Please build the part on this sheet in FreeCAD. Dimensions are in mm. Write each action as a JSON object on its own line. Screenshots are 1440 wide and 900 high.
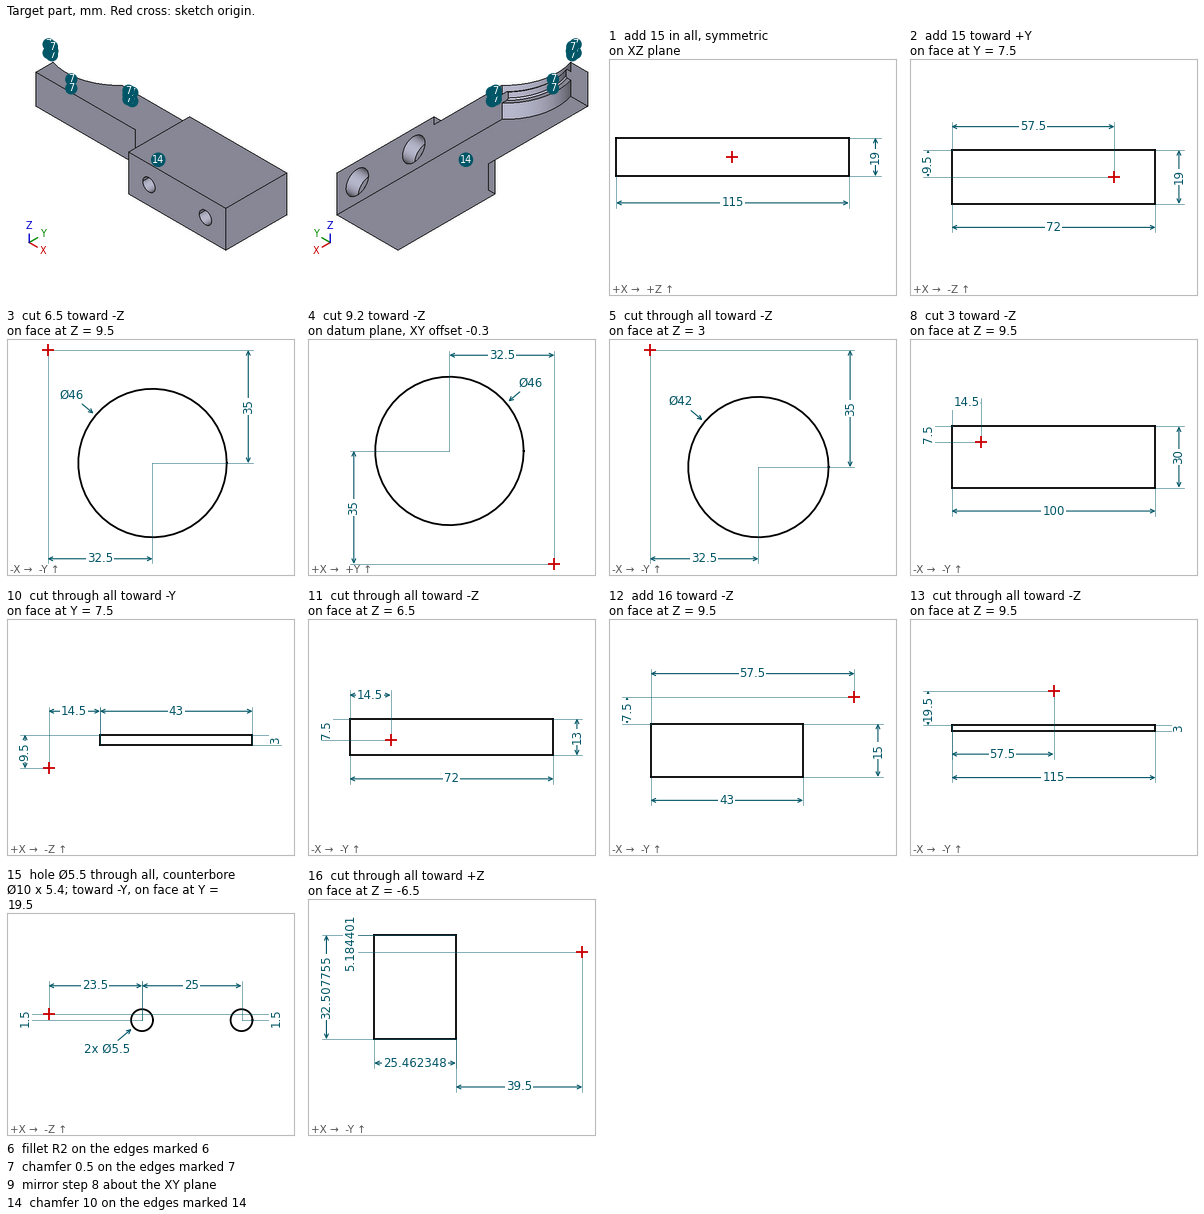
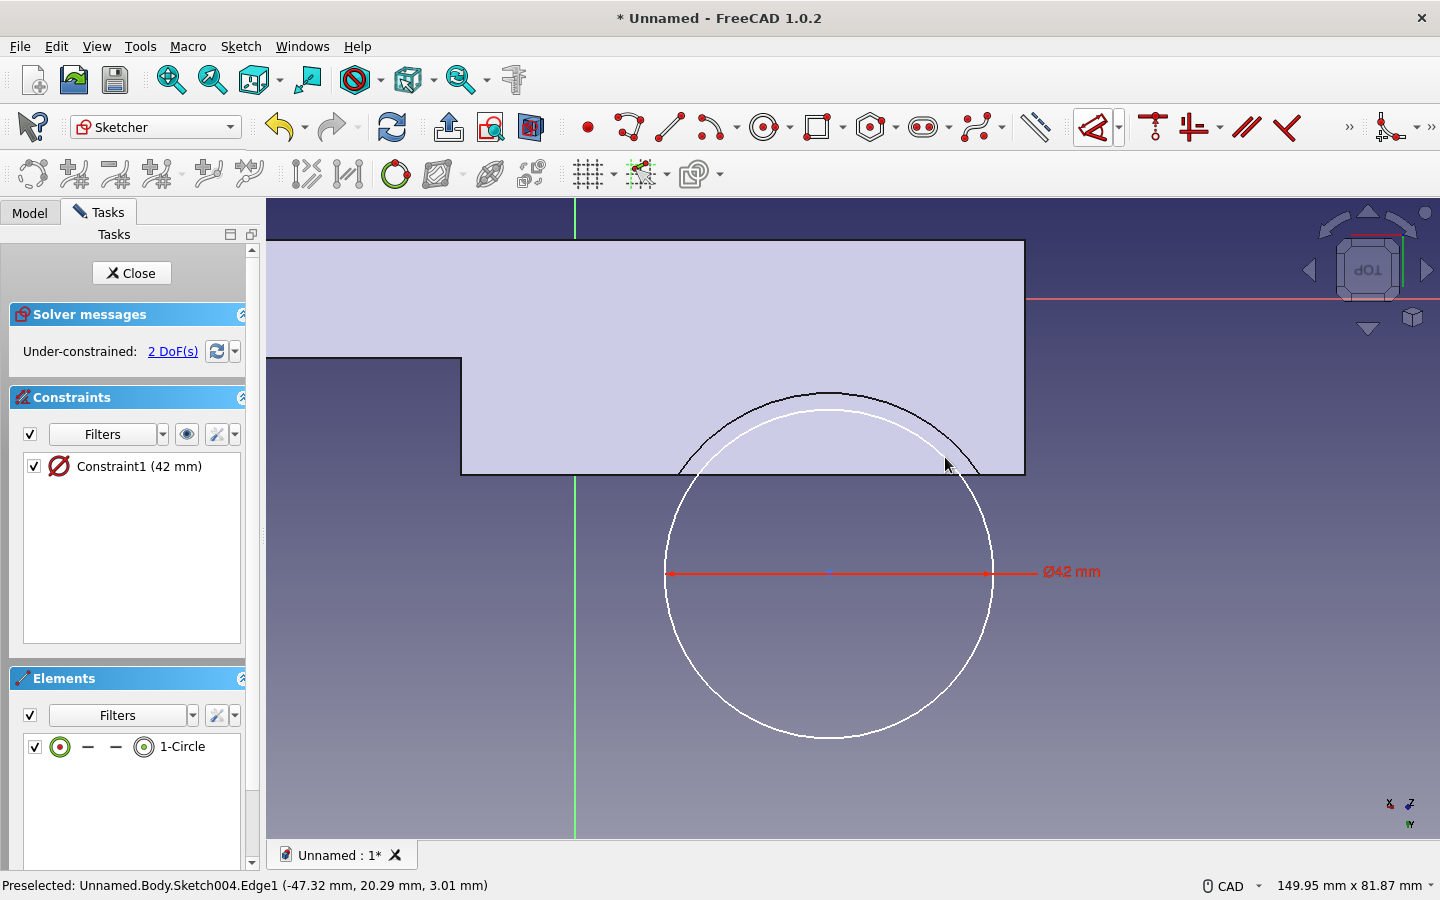
{"action": "left_click", "coordinate": [829, 574]}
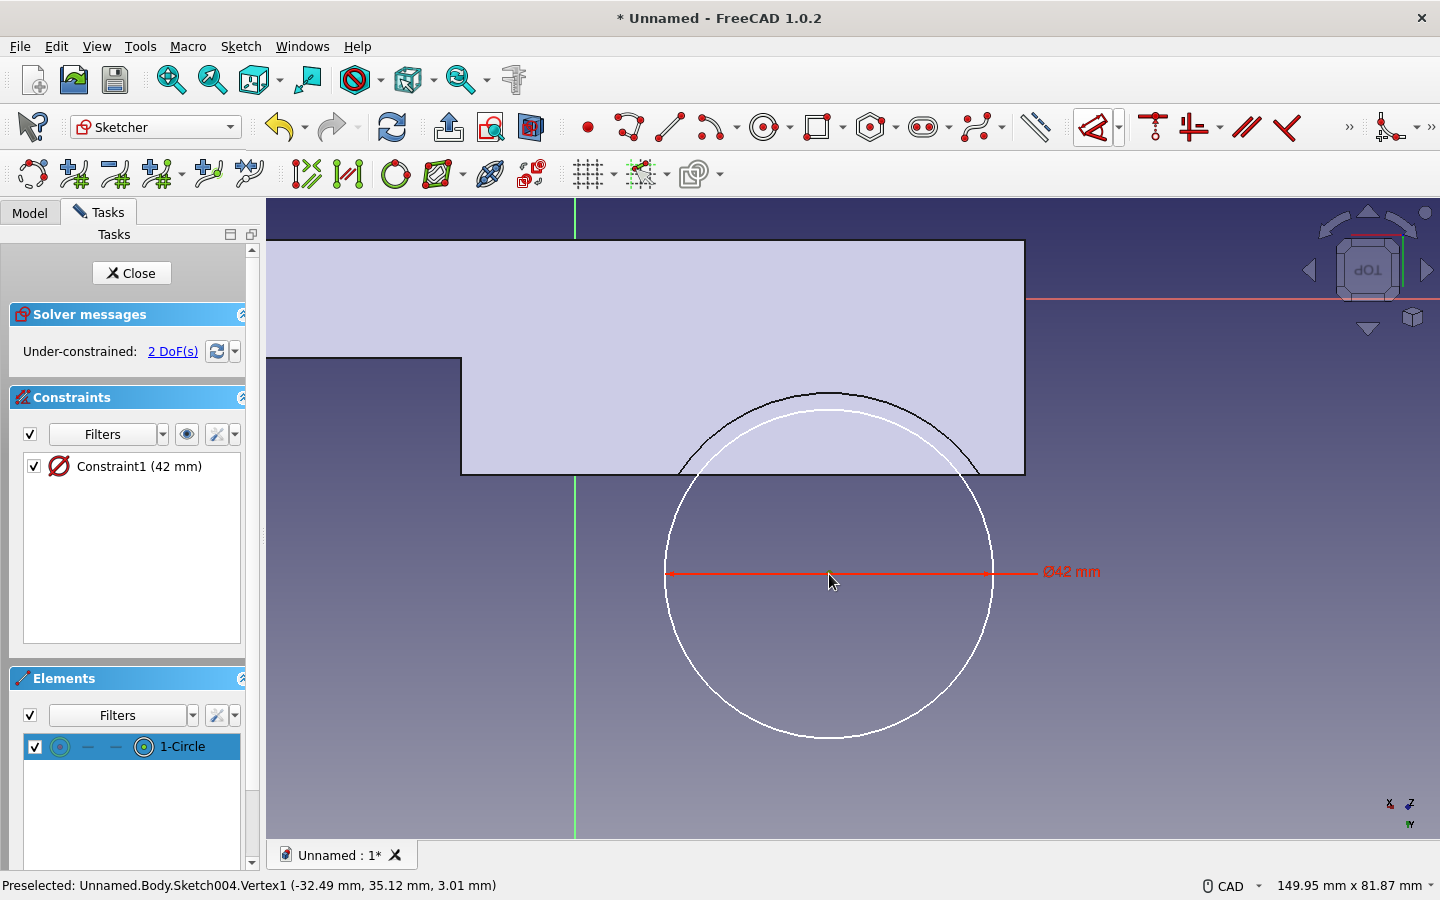
{"action": "left_click", "coordinate": [1118, 128]}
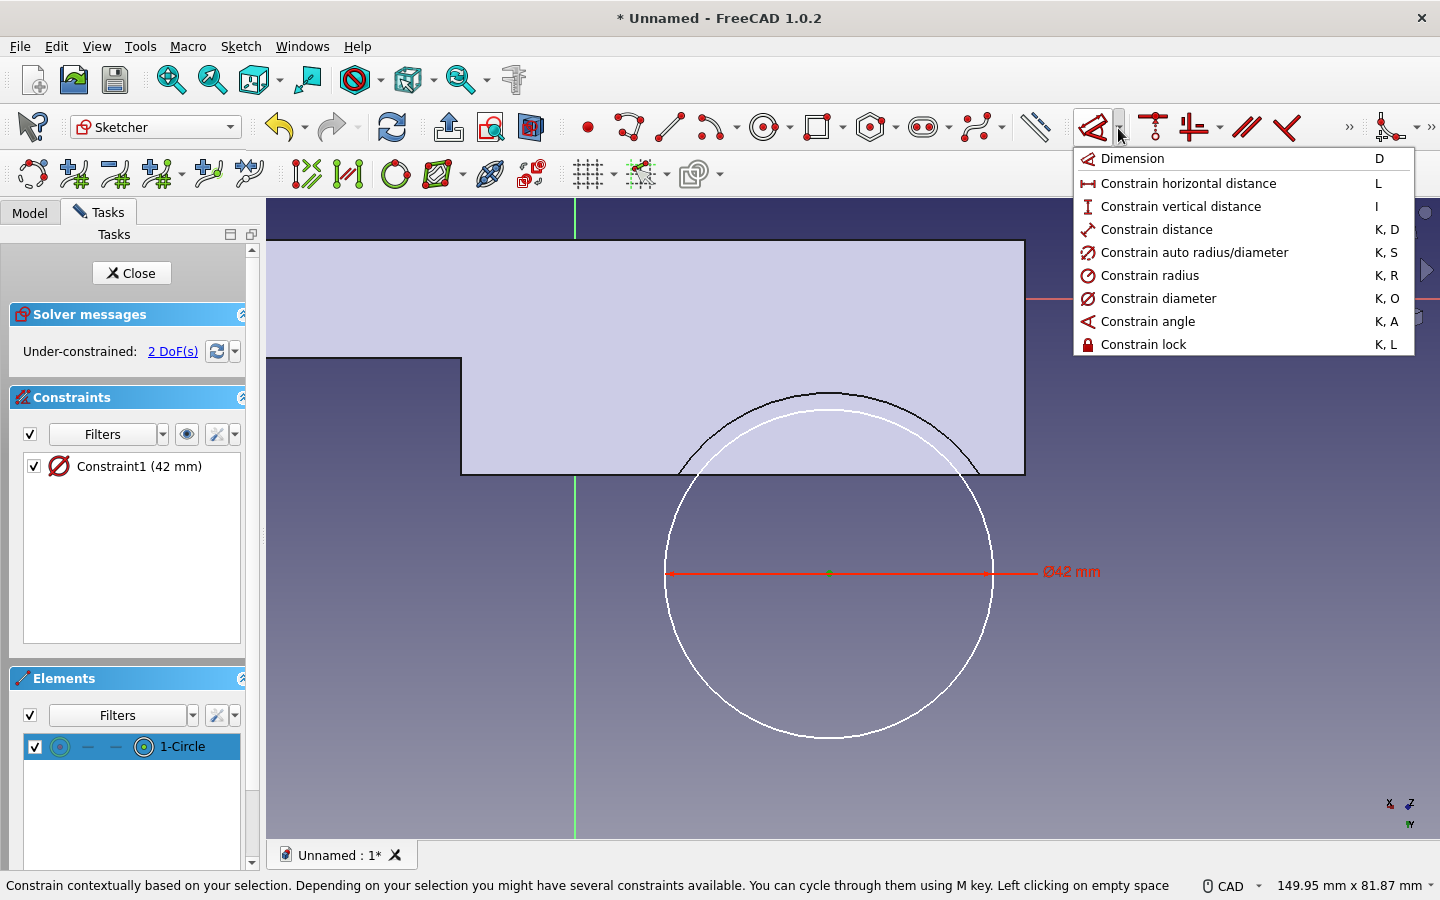
{"action": "left_click", "coordinate": [1244, 206]}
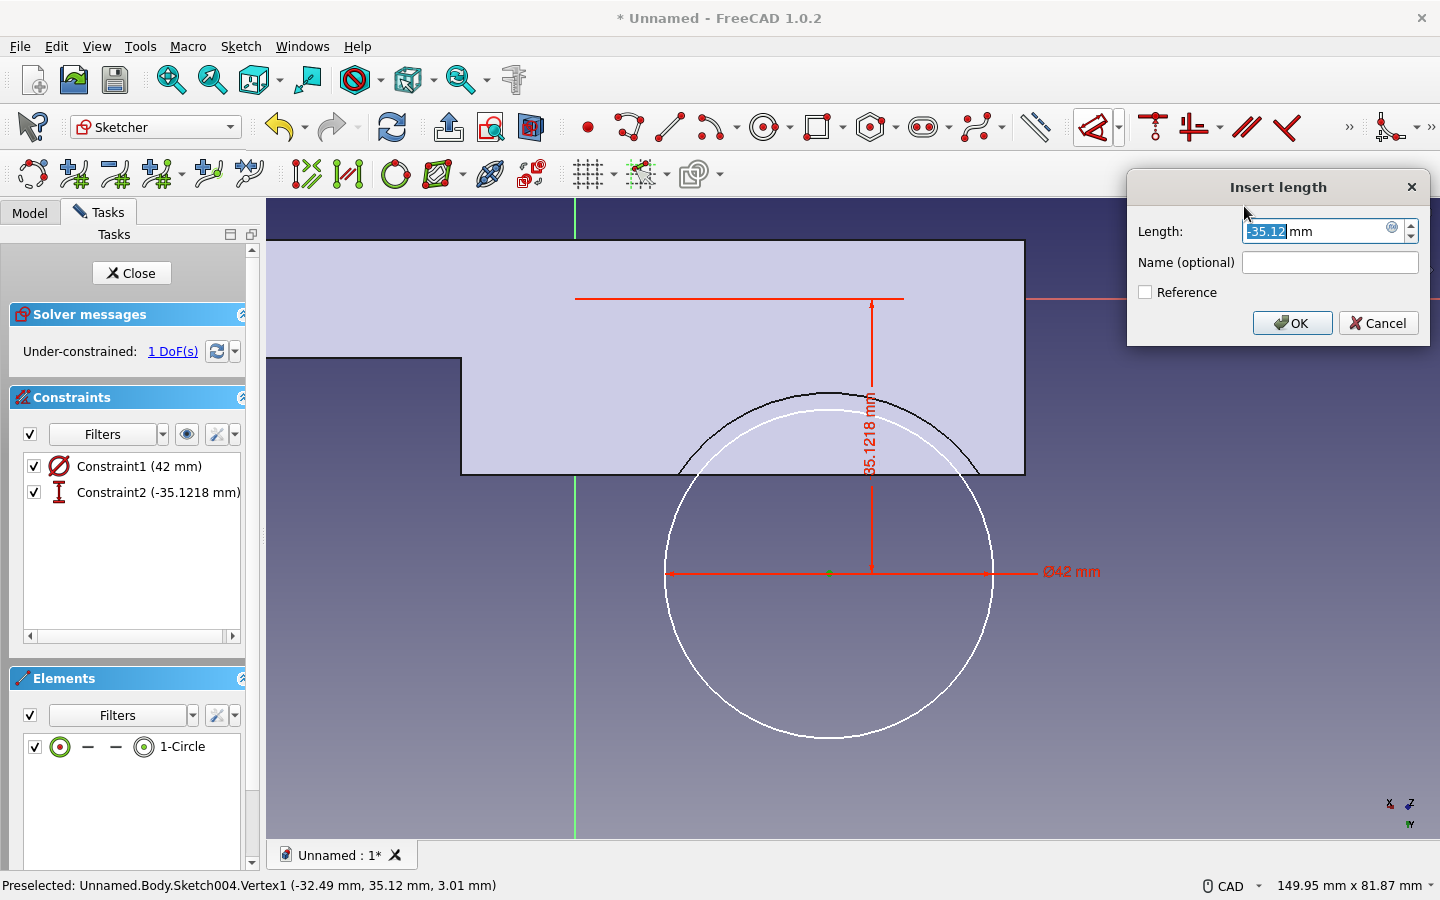
{"action": "type", "text": "-35"}
{"action": "key", "text": "Return"}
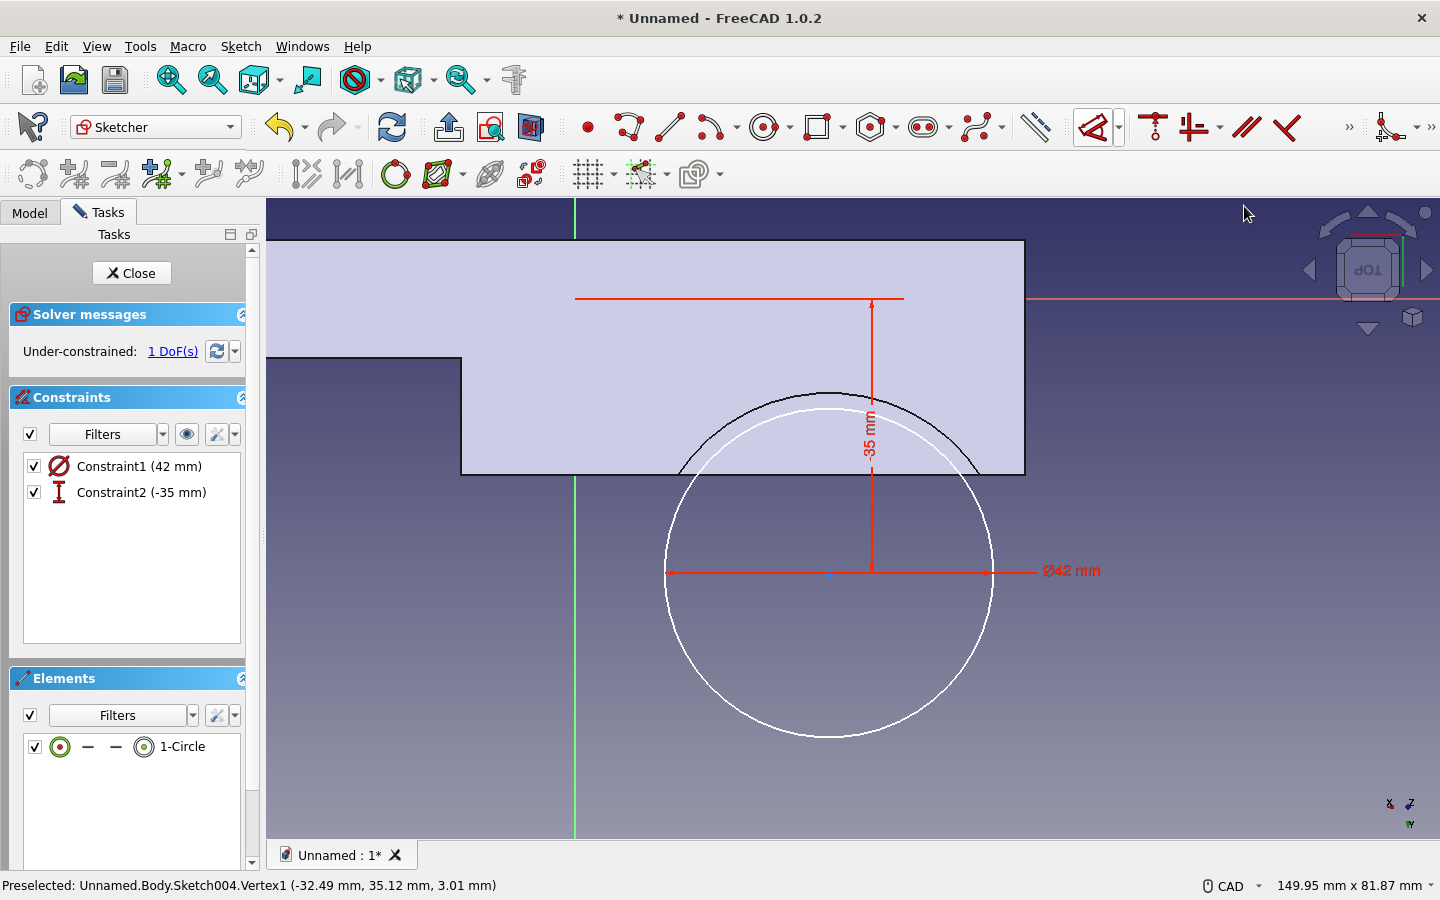
{"action": "left_click", "coordinate": [829, 573]}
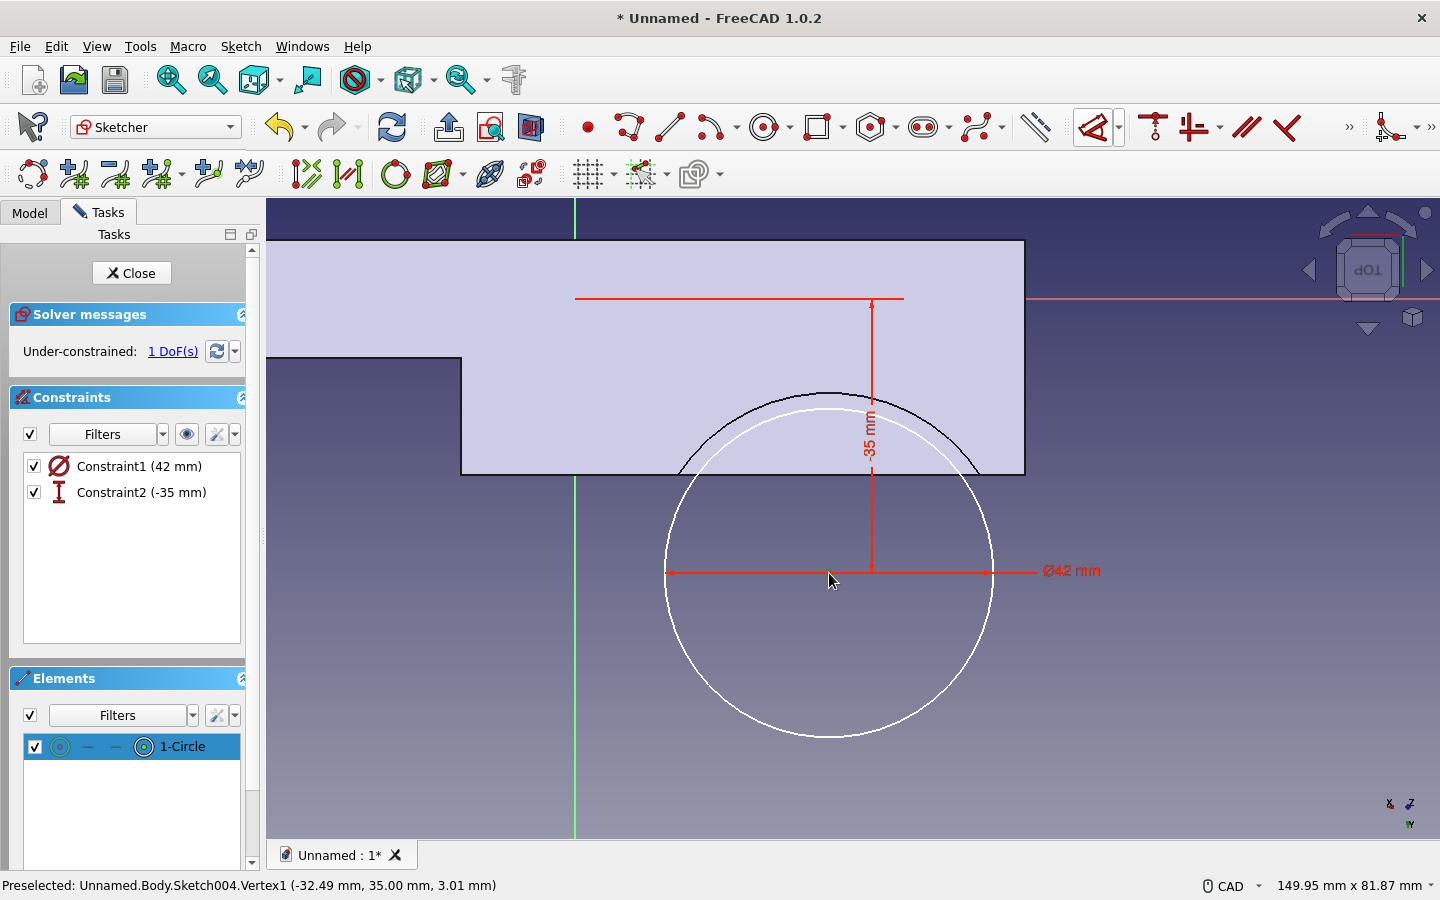
{"action": "key", "text": "l"}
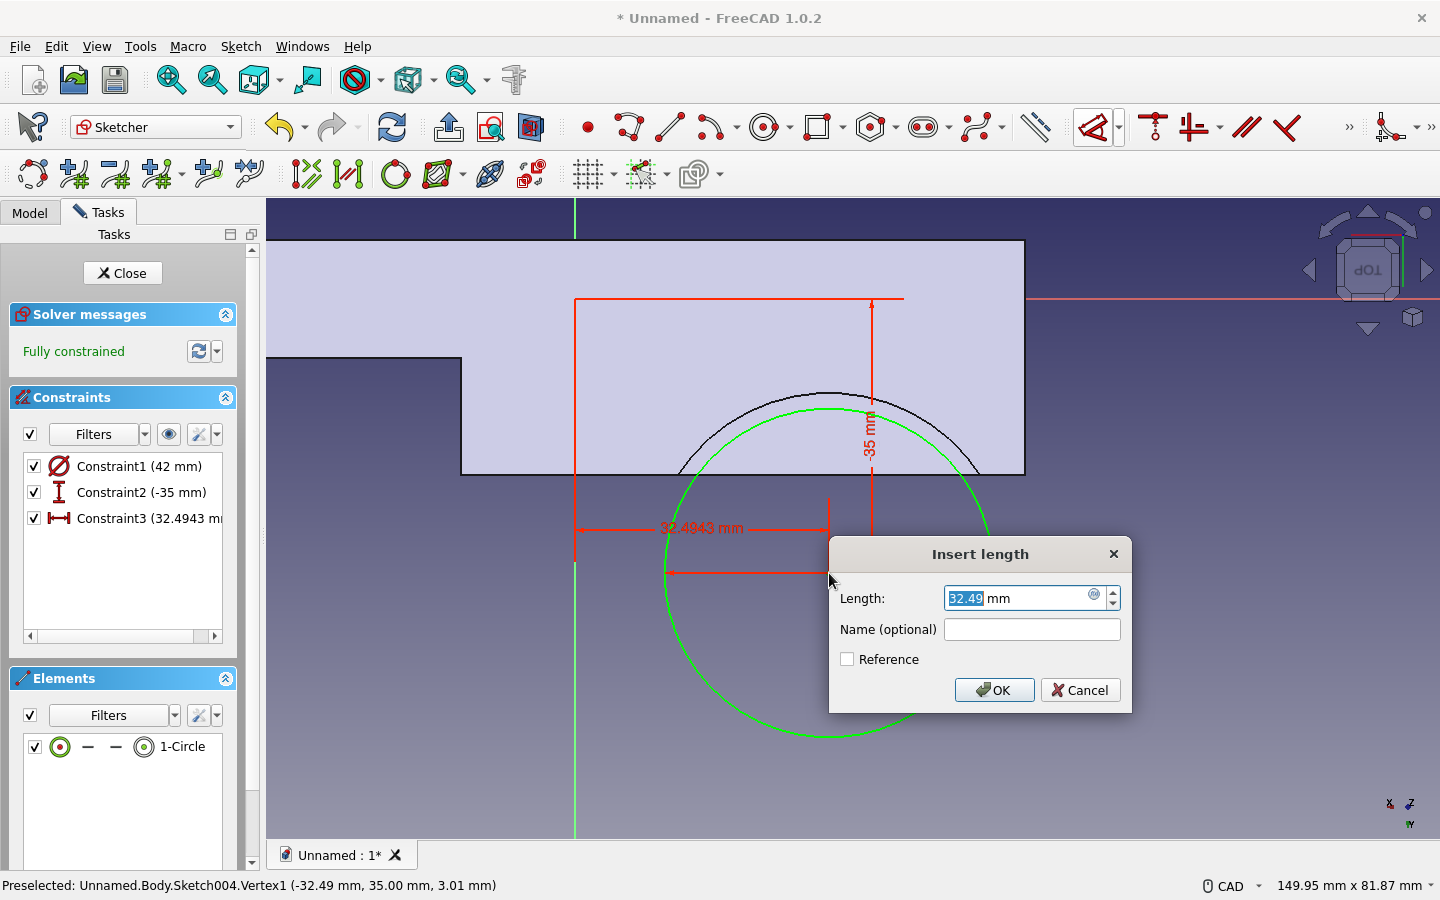
{"action": "type", "text": "32.5"}
{"action": "key", "text": "Return"}